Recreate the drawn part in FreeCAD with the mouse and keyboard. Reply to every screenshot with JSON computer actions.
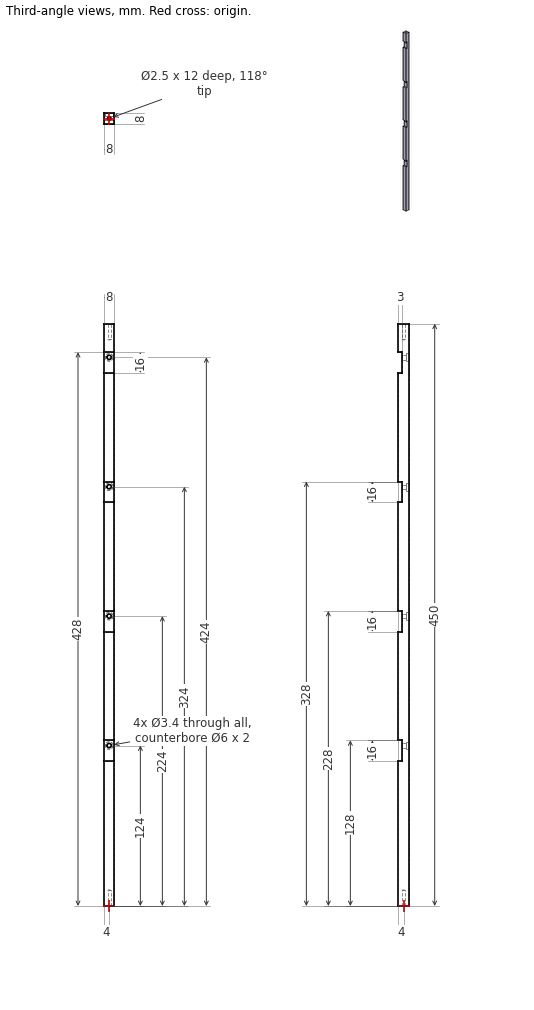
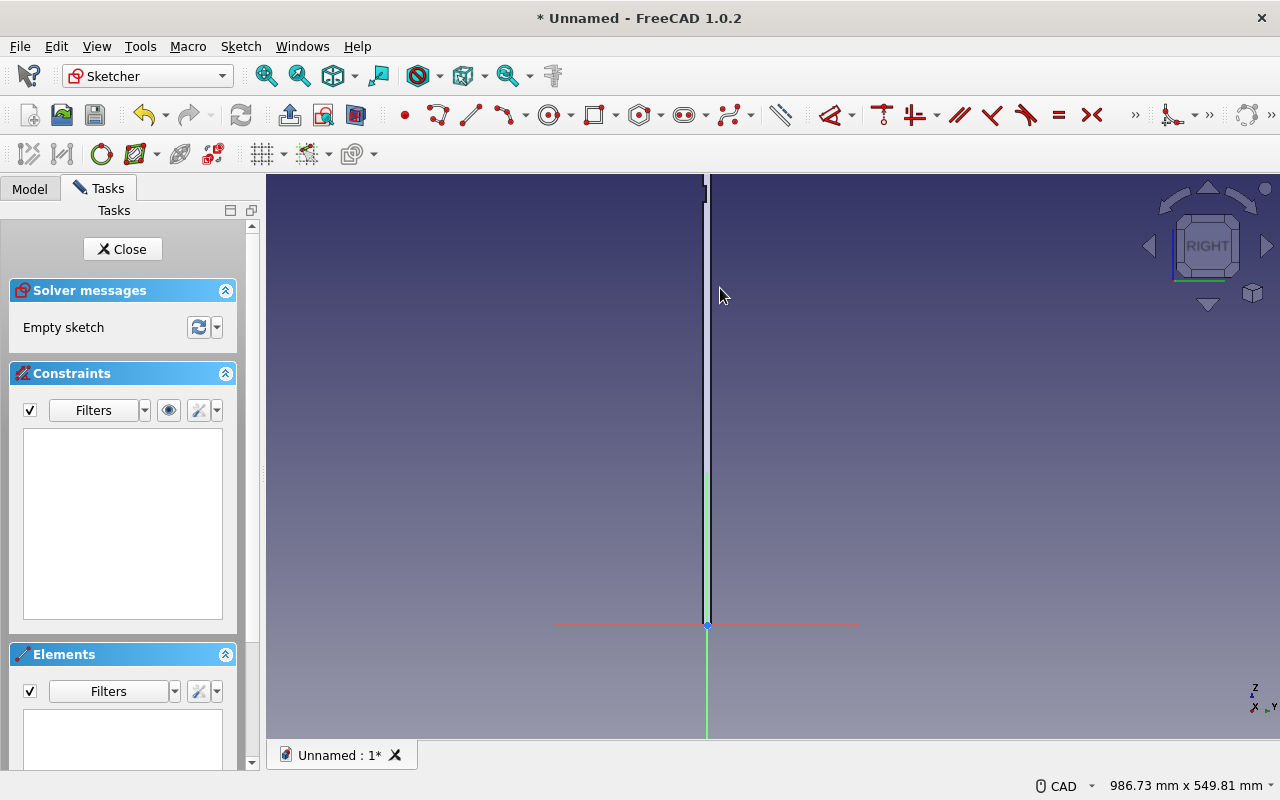
{"action": "key", "text": "g r"}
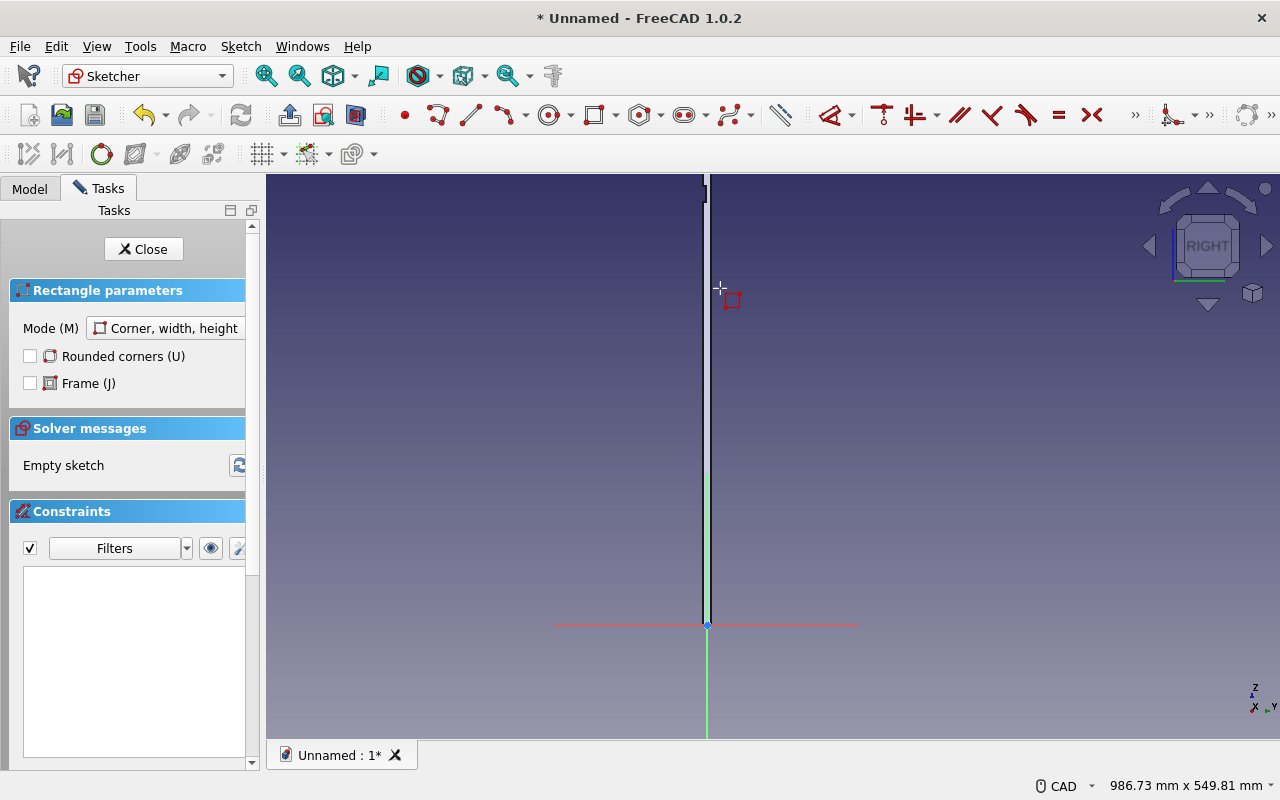
{"action": "scroll", "coordinate": [703, 288], "scroll_direction": "up", "scroll_amount": 9}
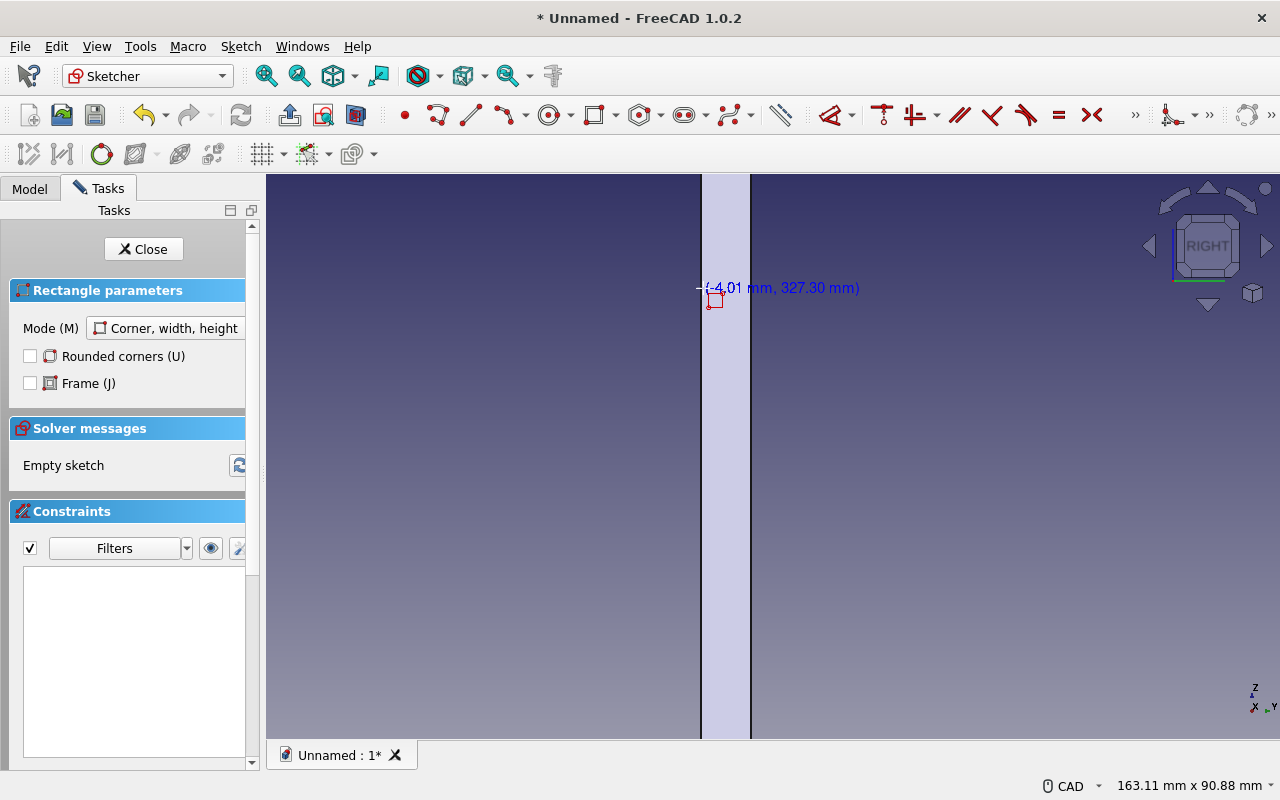
{"action": "left_click", "coordinate": [701, 289]}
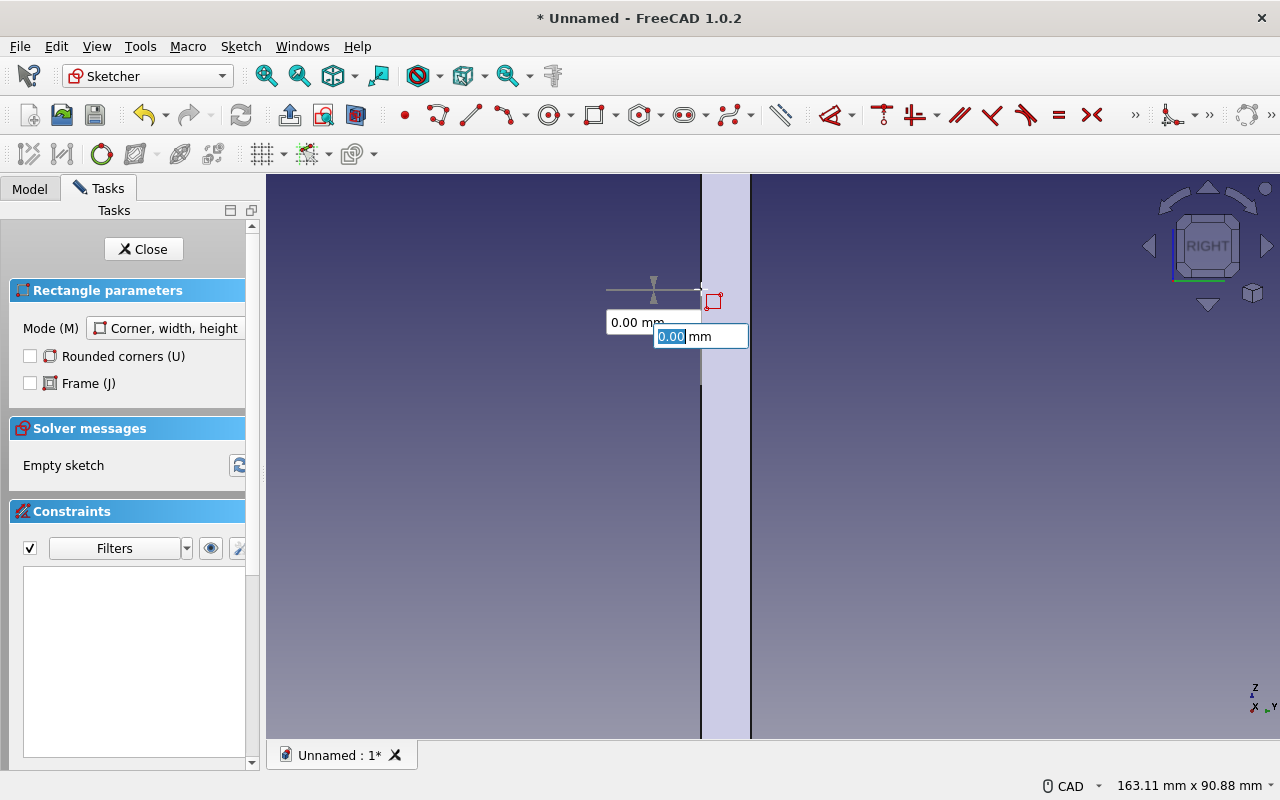
{"action": "scroll", "coordinate": [720, 388], "scroll_direction": "up", "scroll_amount": 5}
{"action": "mouse_move", "coordinate": [718, 388]}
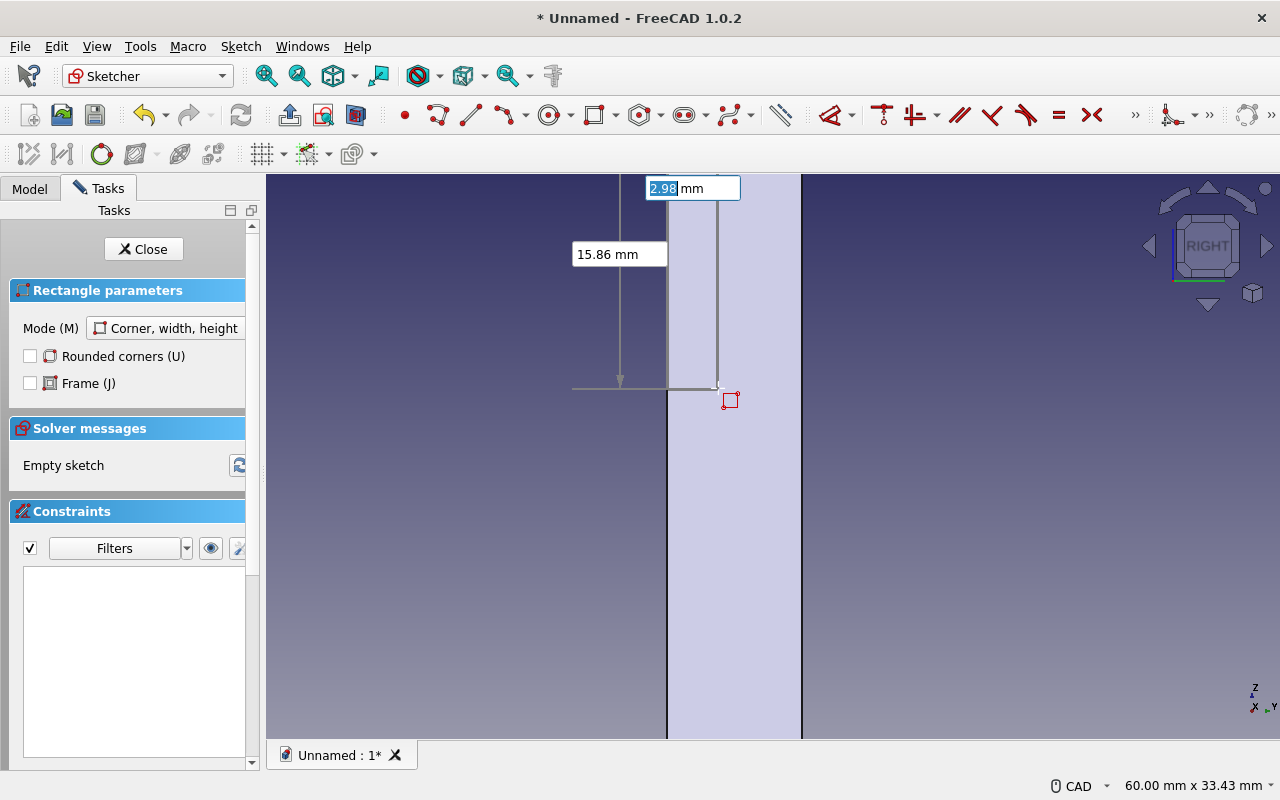
{"action": "type", "text": "3"}
{"action": "key", "text": "Tab"}
{"action": "type", "text": "16"}
{"action": "key", "text": "Return"}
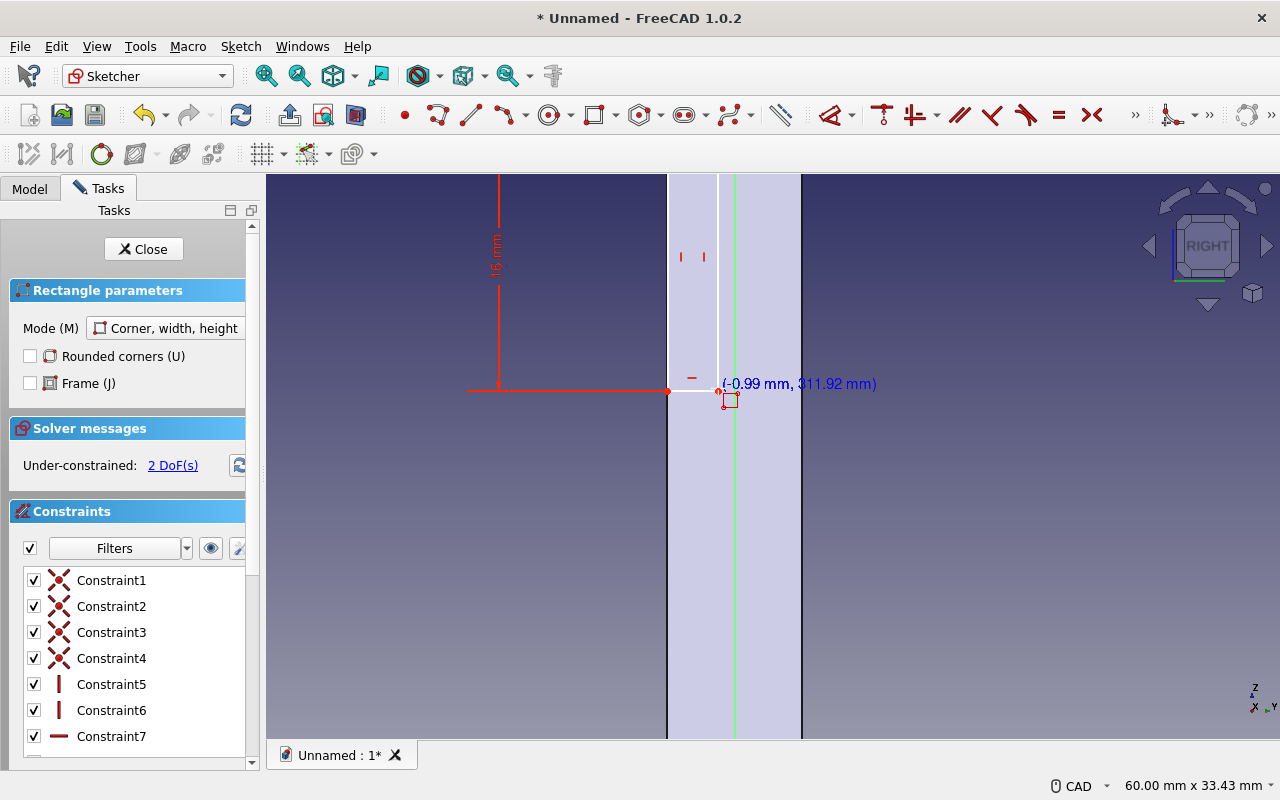
{"action": "scroll", "coordinate": [705, 299], "scroll_direction": "down", "scroll_amount": 14}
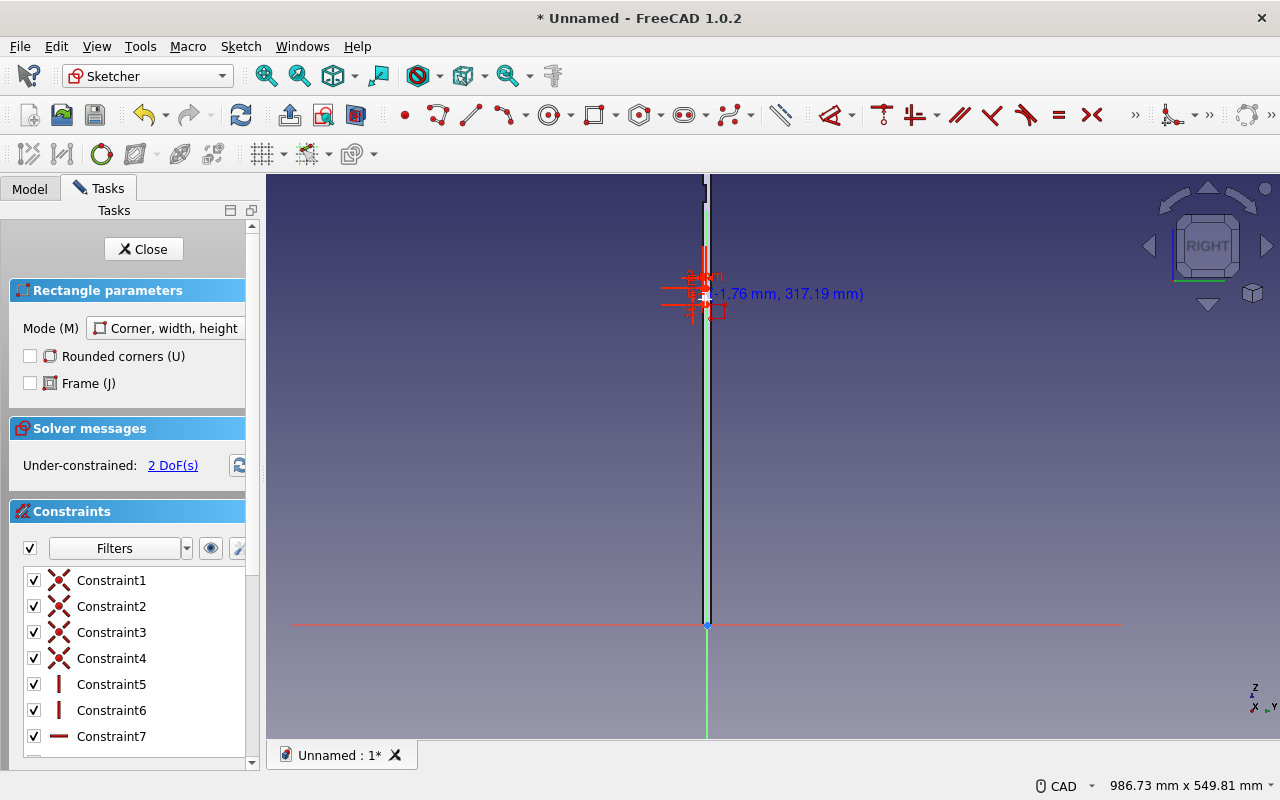
{"action": "scroll", "coordinate": [703, 391], "scroll_direction": "up", "scroll_amount": 9}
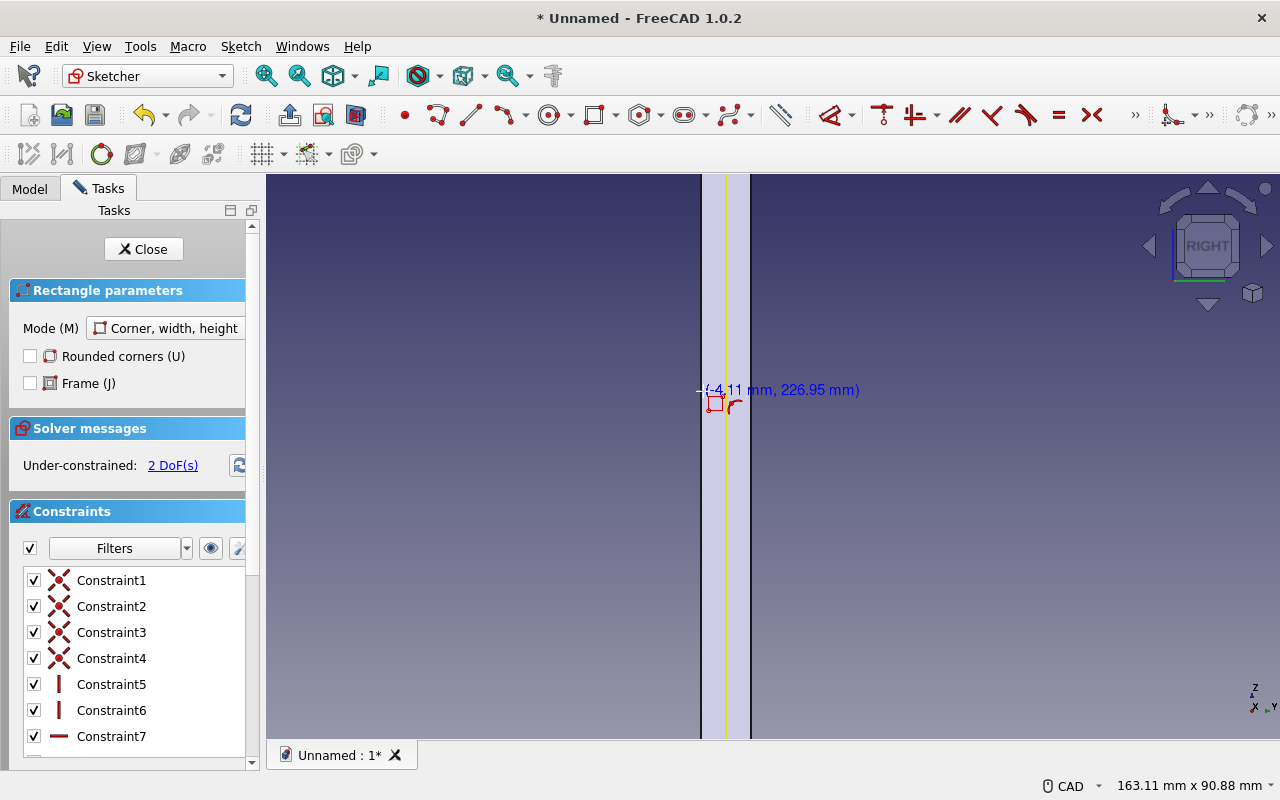
{"action": "left_click", "coordinate": [701, 389]}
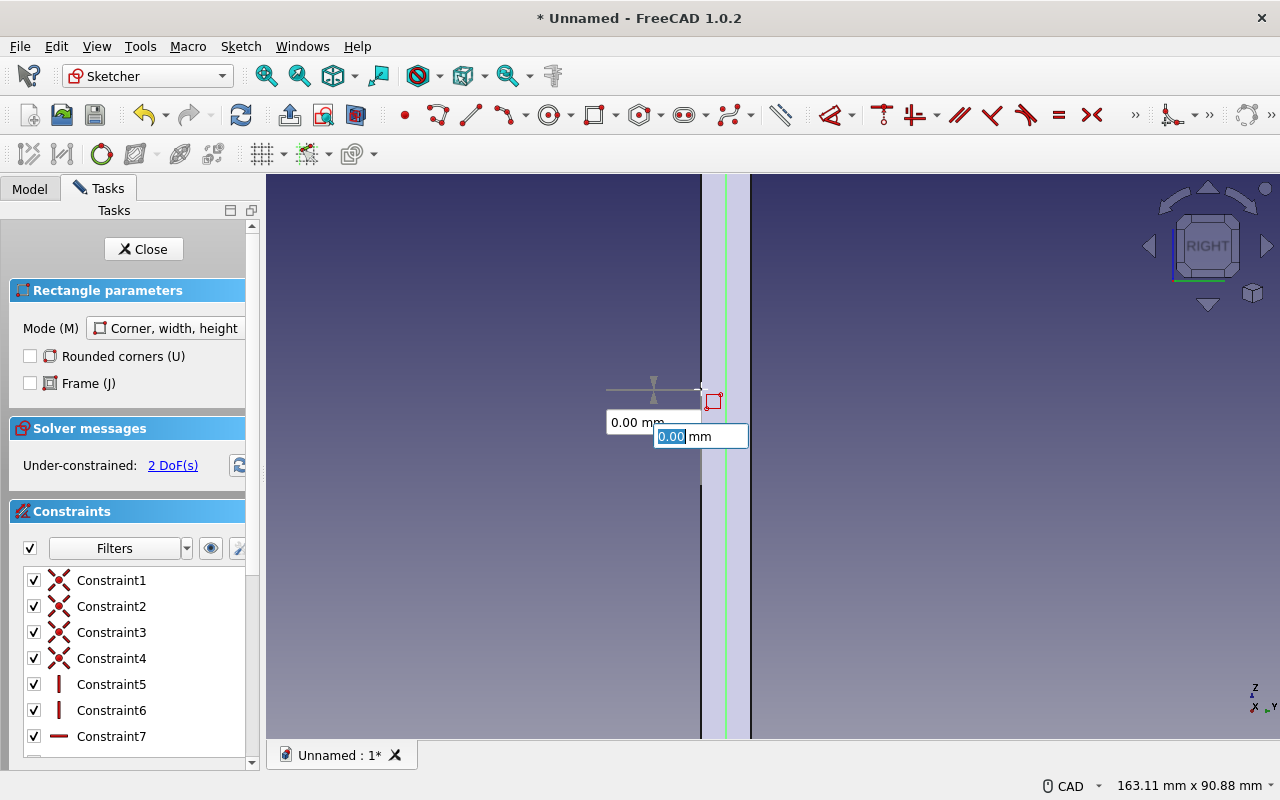
{"action": "scroll", "coordinate": [720, 488], "scroll_direction": "up", "scroll_amount": 5}
{"action": "mouse_move", "coordinate": [720, 487]}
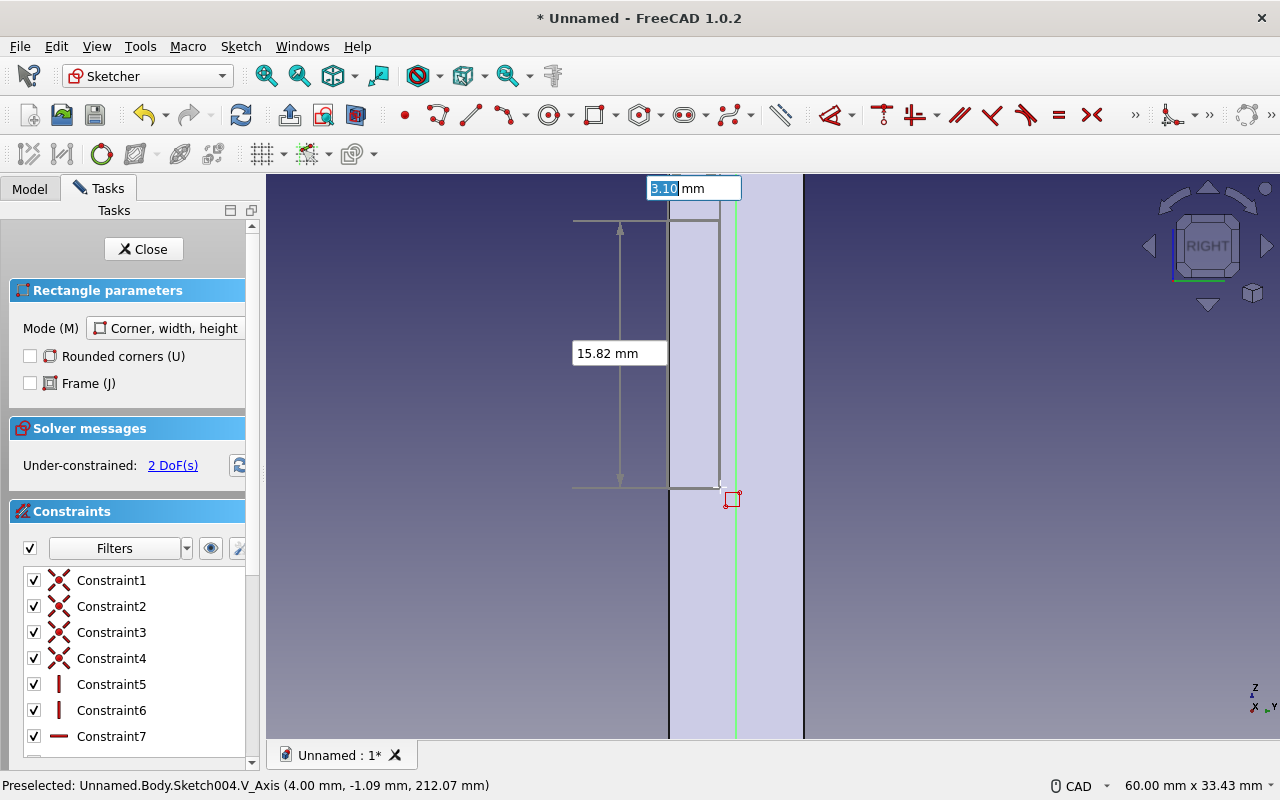
{"action": "type", "text": "3"}
{"action": "key", "text": "Tab"}
{"action": "type", "text": "16"}
{"action": "key", "text": "Return"}